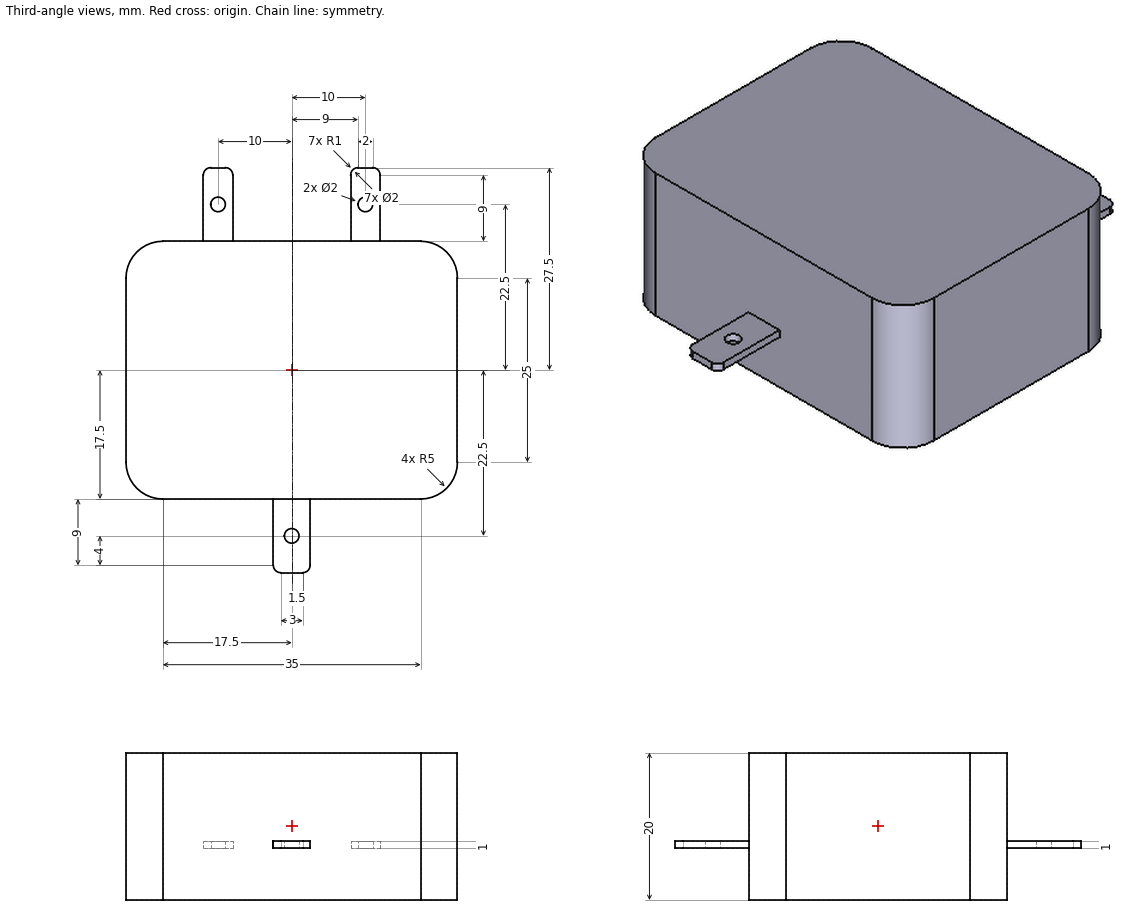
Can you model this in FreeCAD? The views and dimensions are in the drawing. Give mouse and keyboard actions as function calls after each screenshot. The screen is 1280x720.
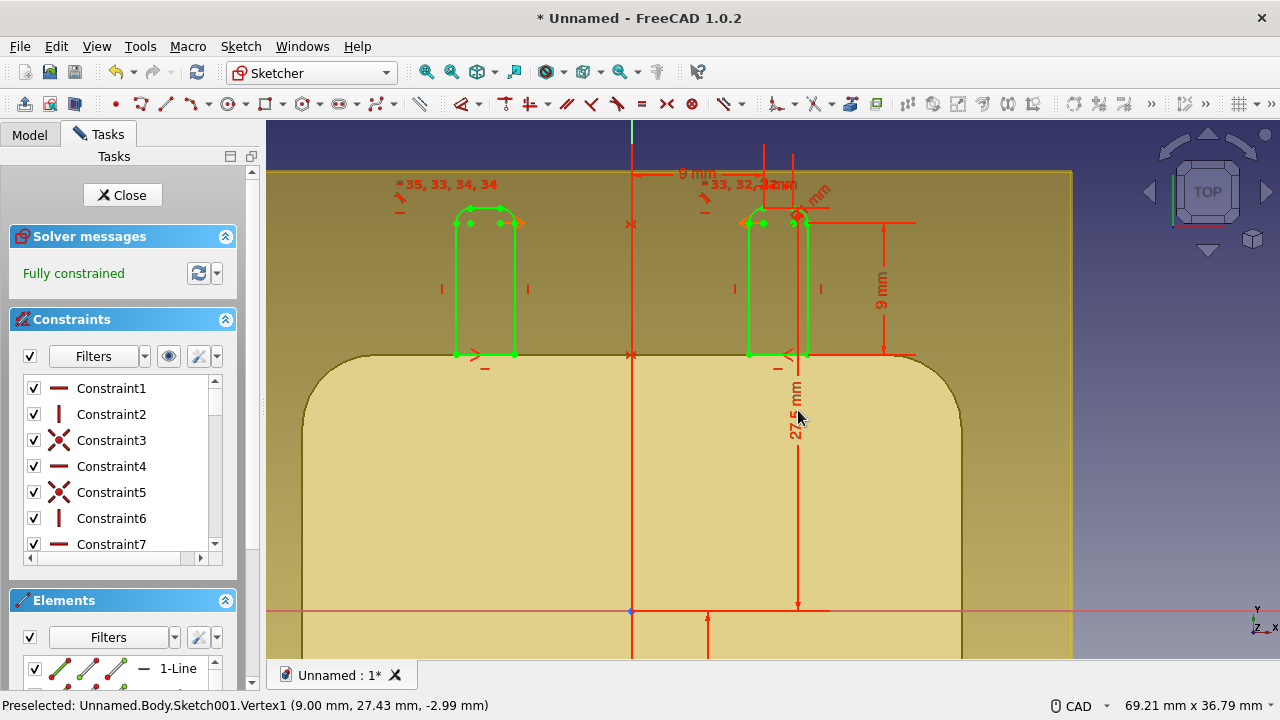
click(123, 195)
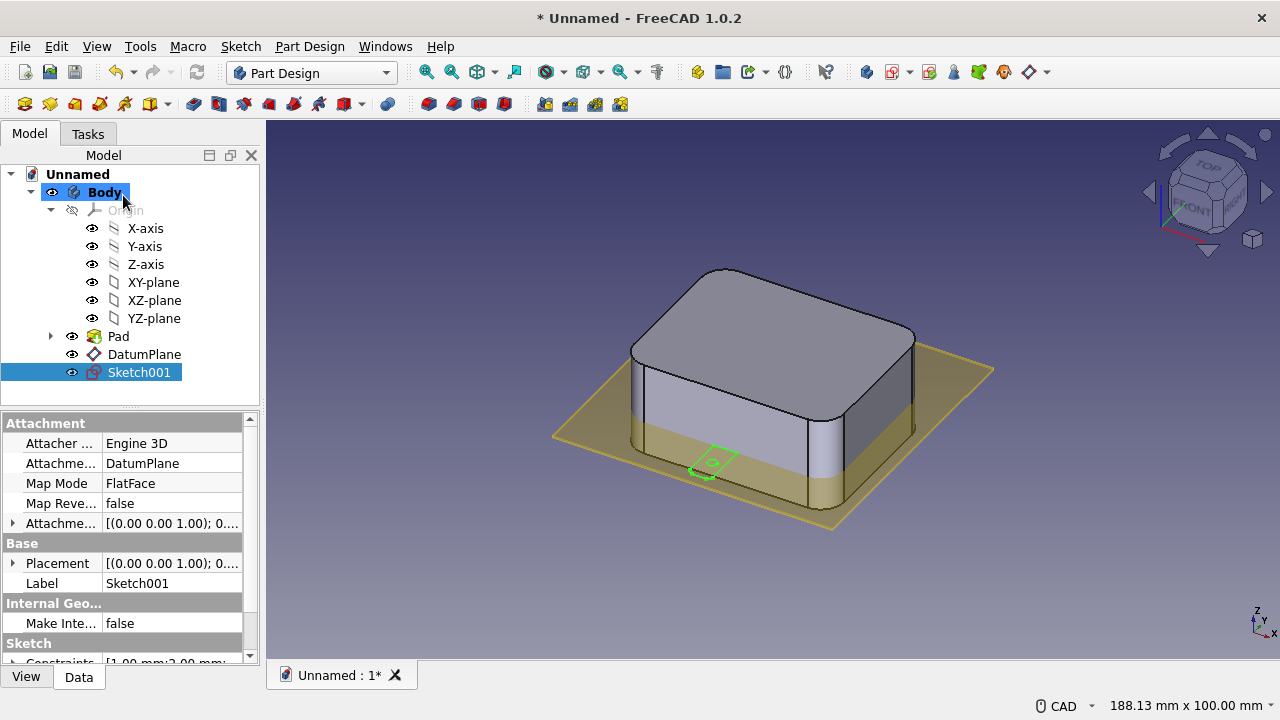
click(25, 104)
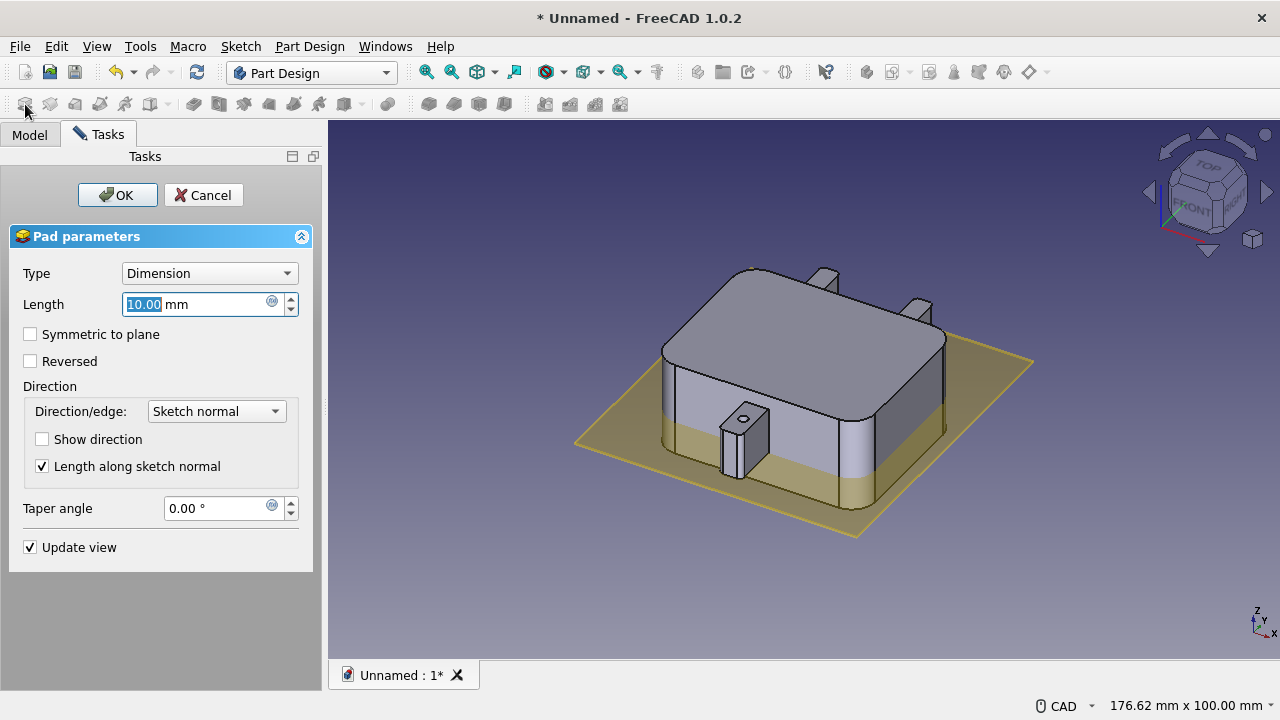
text(1)
key(Tab)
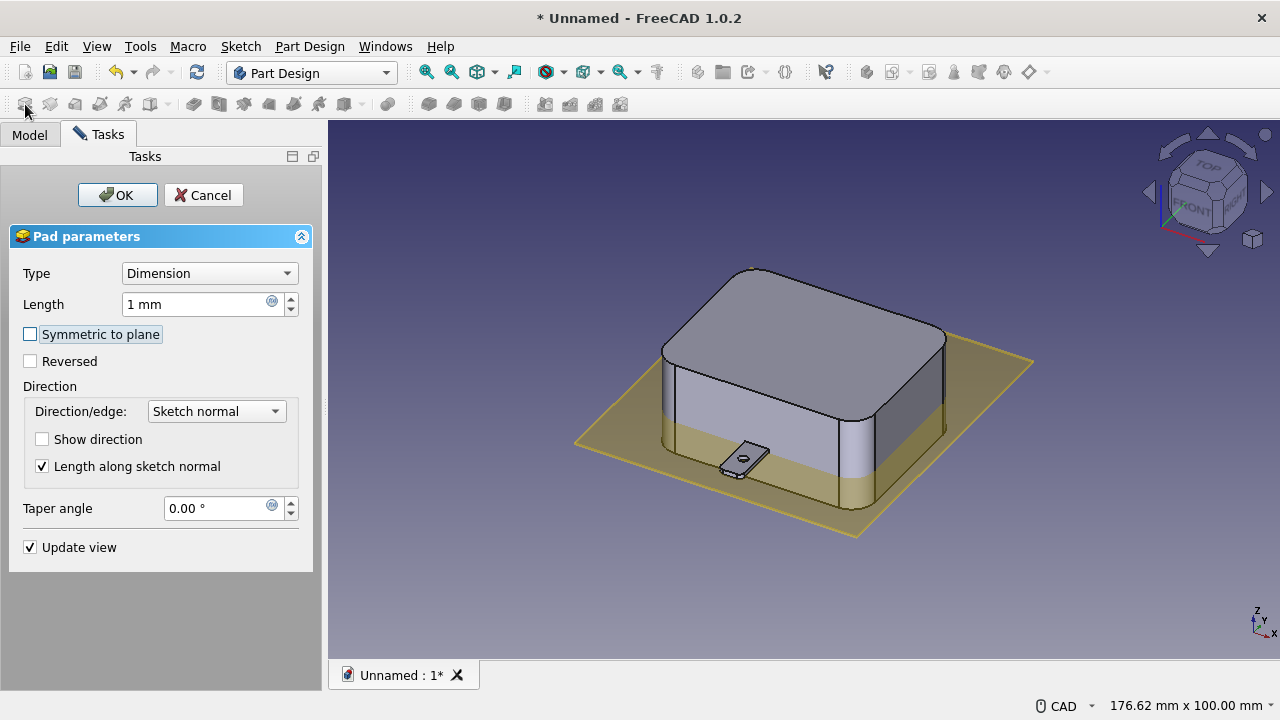
click(118, 195)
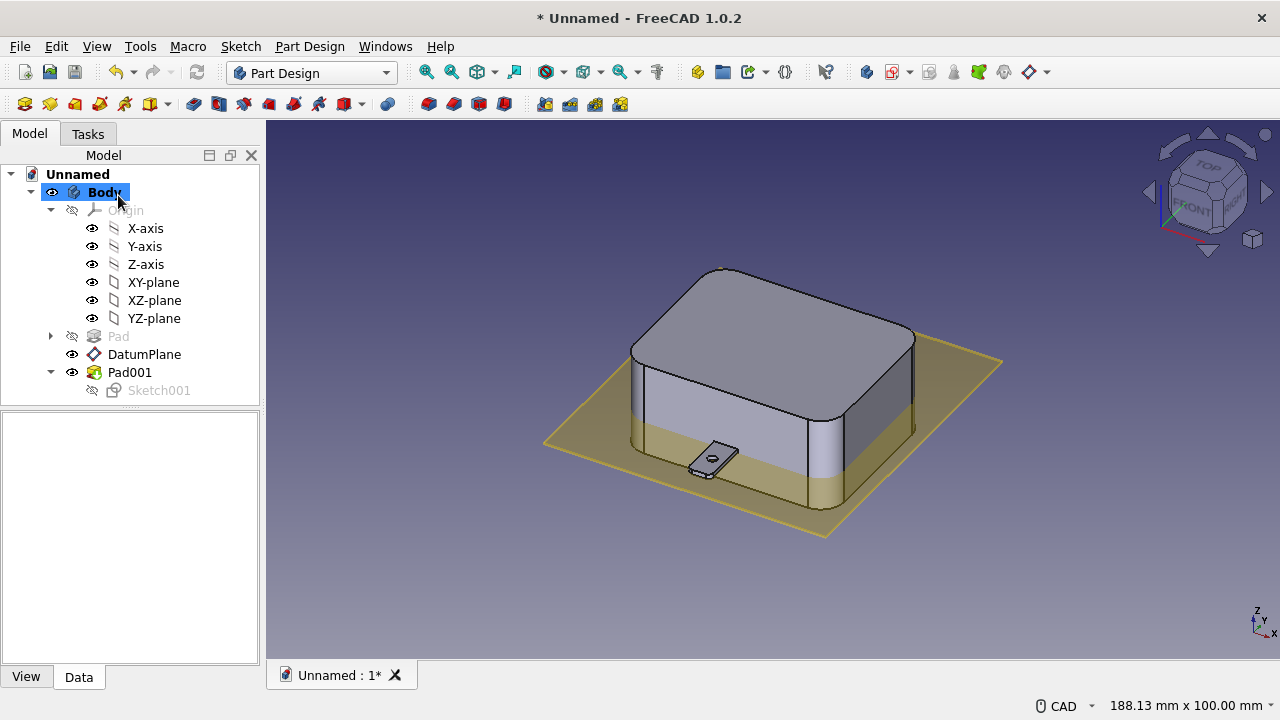
click(117, 354)
key(space)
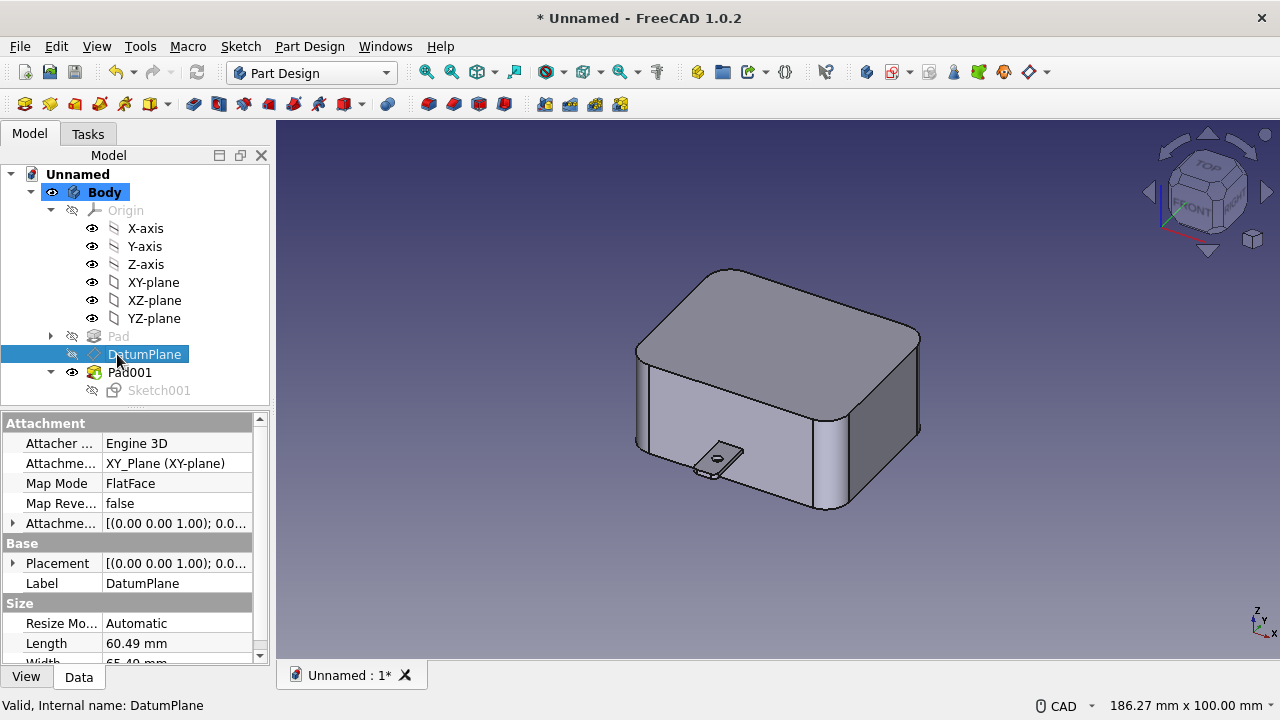
key(5)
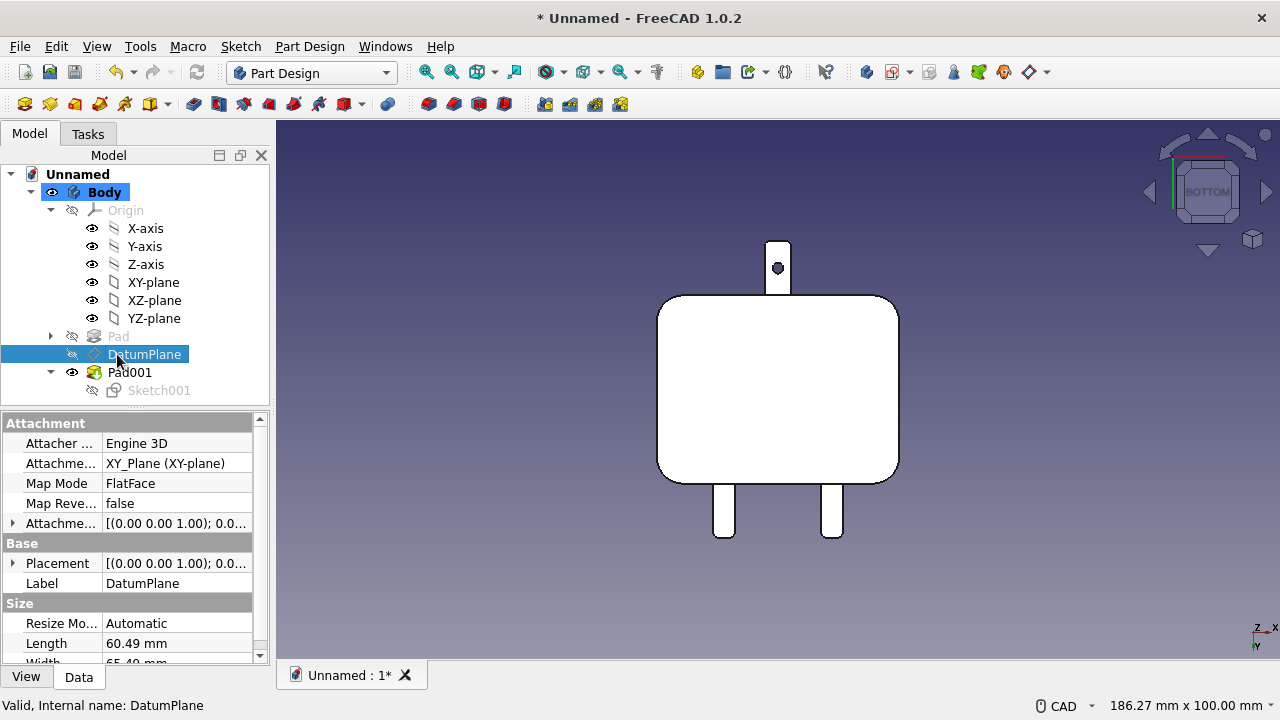
click(778, 252)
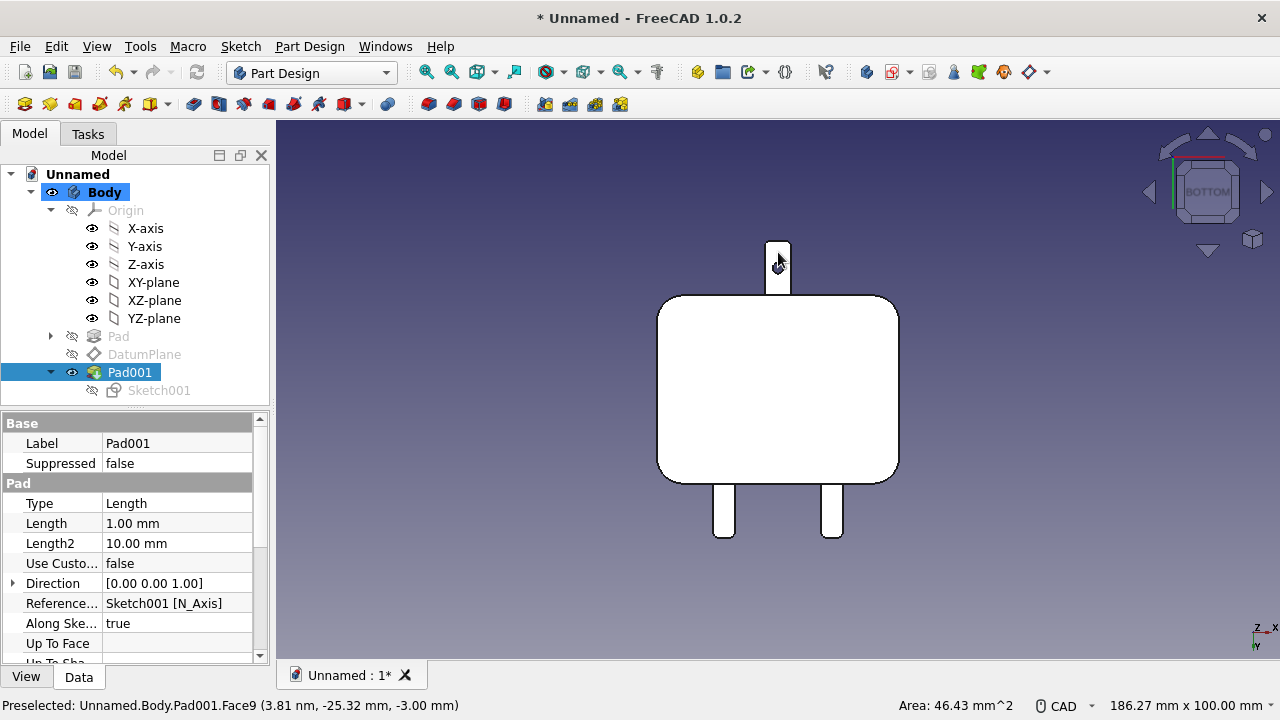
click(892, 72)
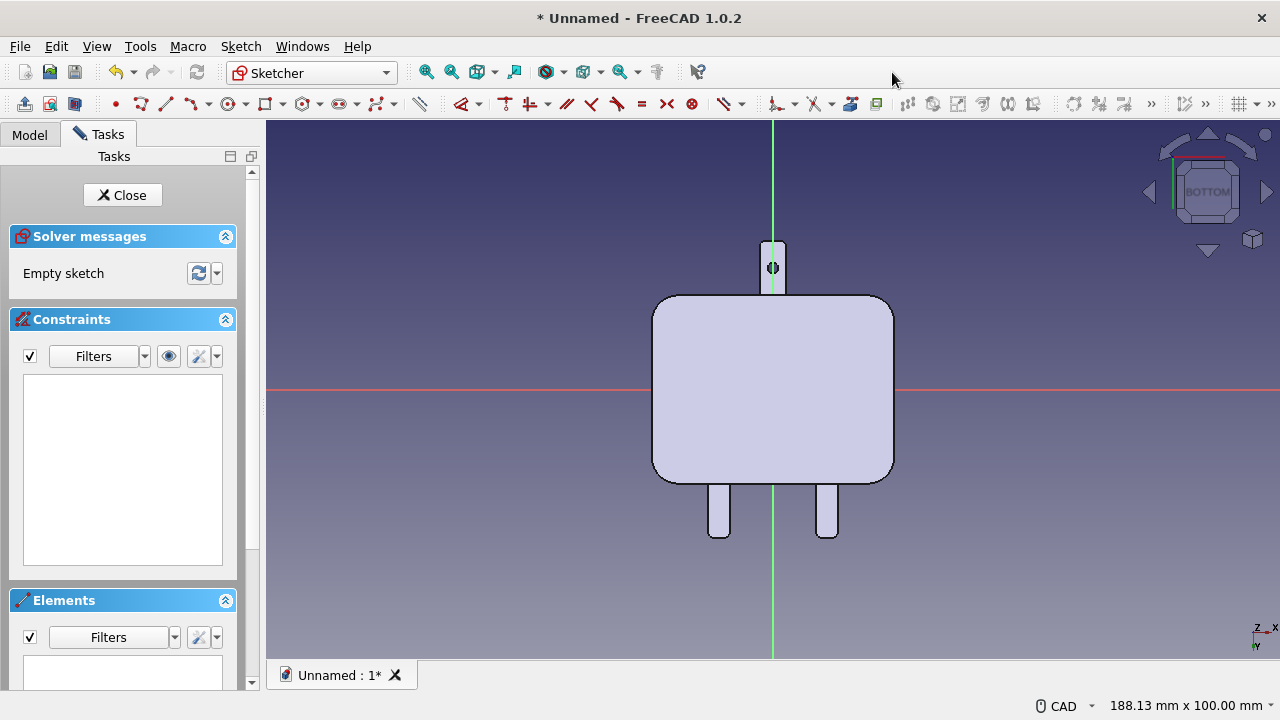
scroll(813, 490, up, 5)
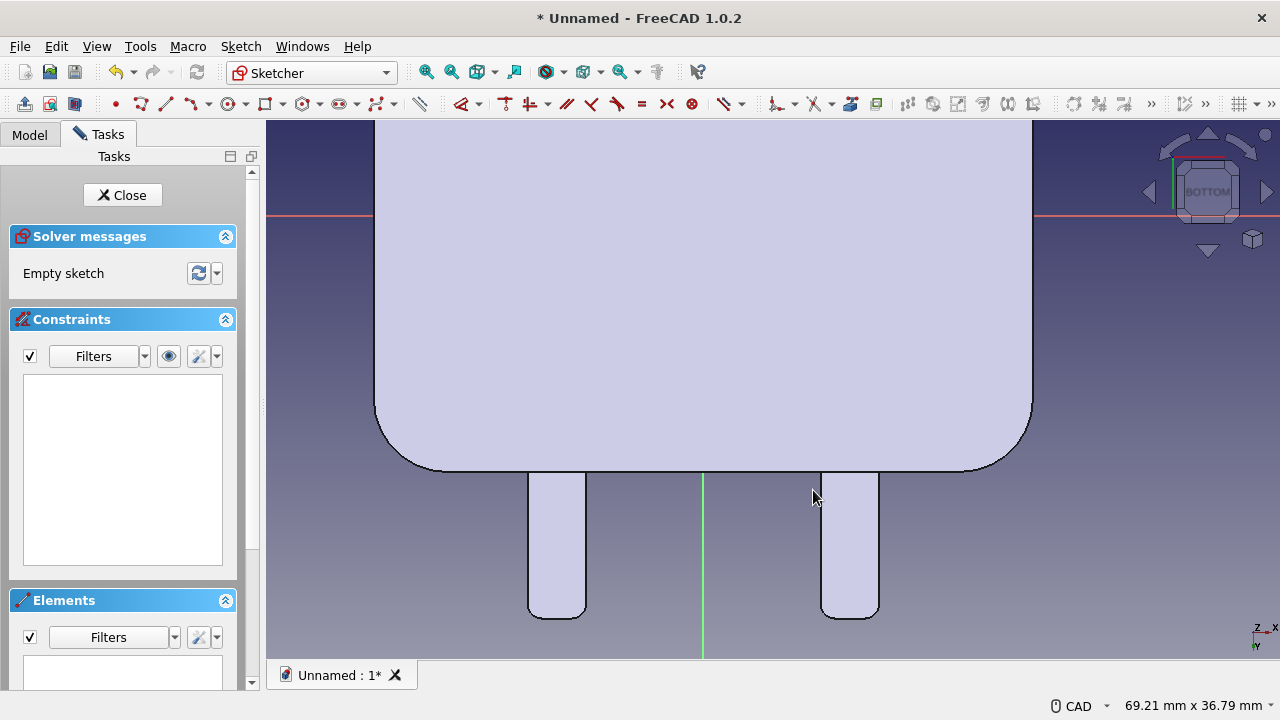
key(g)
key(c)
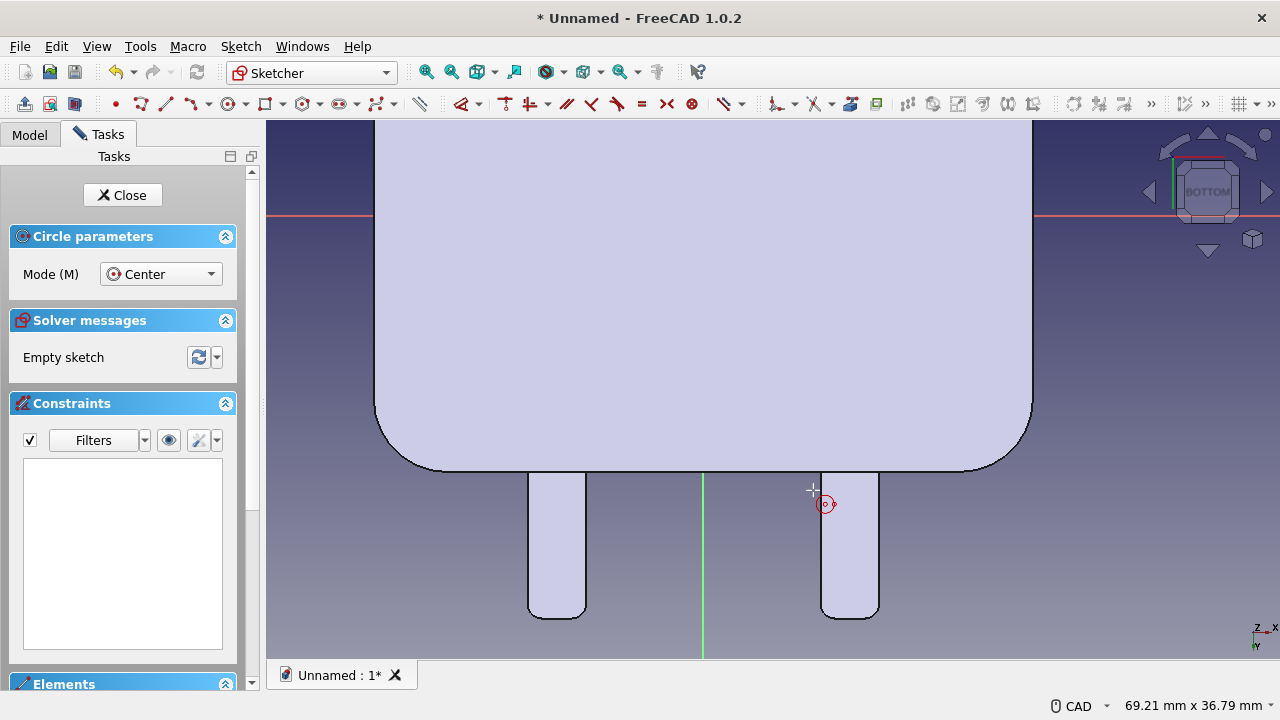
scroll(850, 545, up, 3)